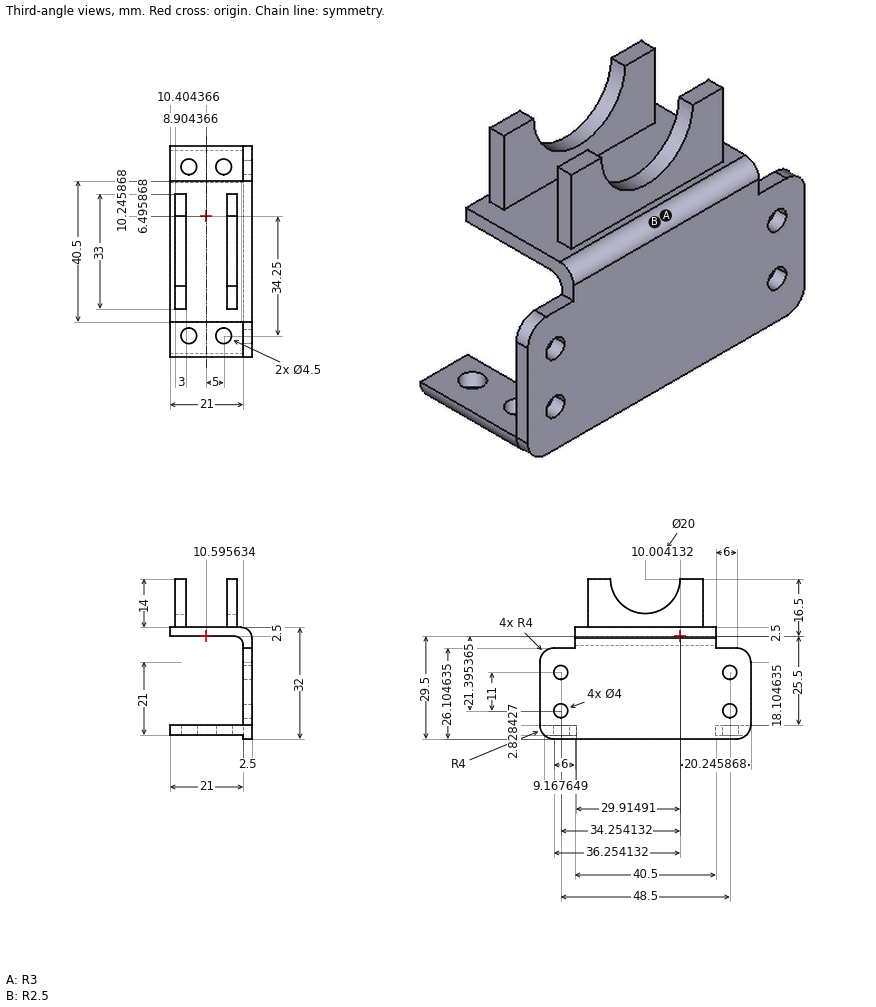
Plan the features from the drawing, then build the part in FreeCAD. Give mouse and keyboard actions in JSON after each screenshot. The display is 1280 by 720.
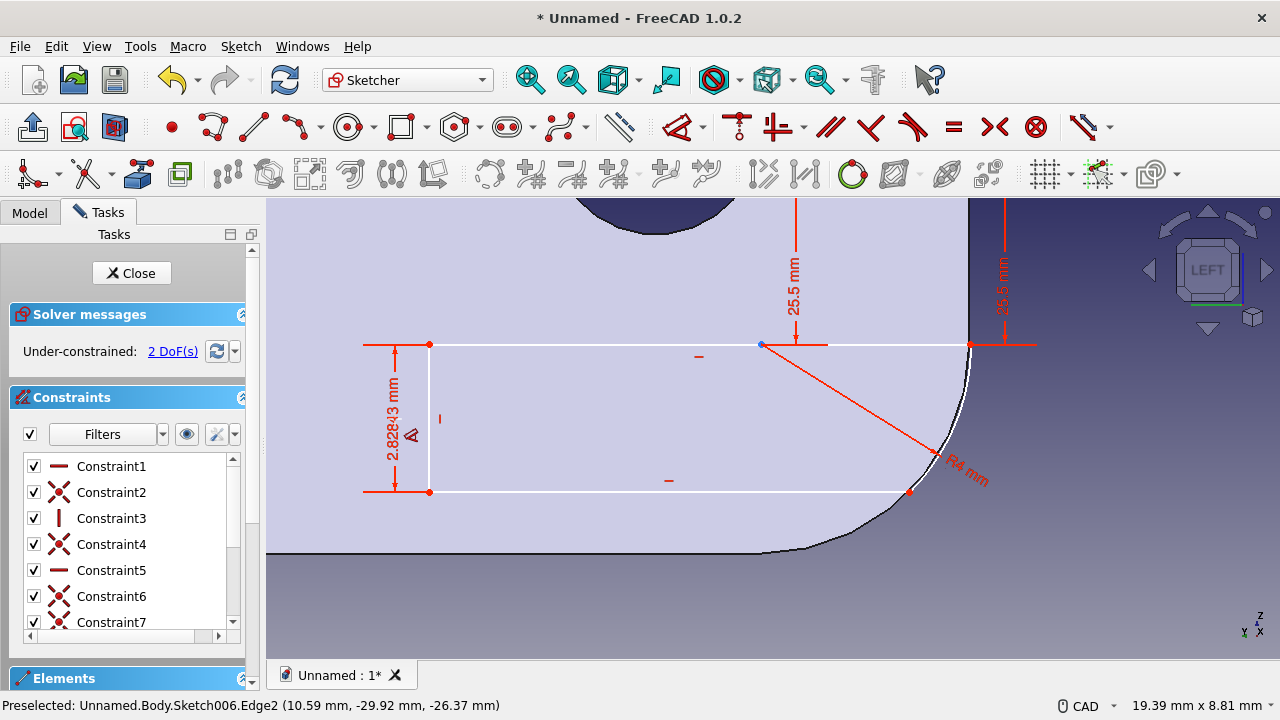
{"action": "left_click", "coordinate": [573, 492]}
{"action": "left_click", "coordinate": [669, 526]}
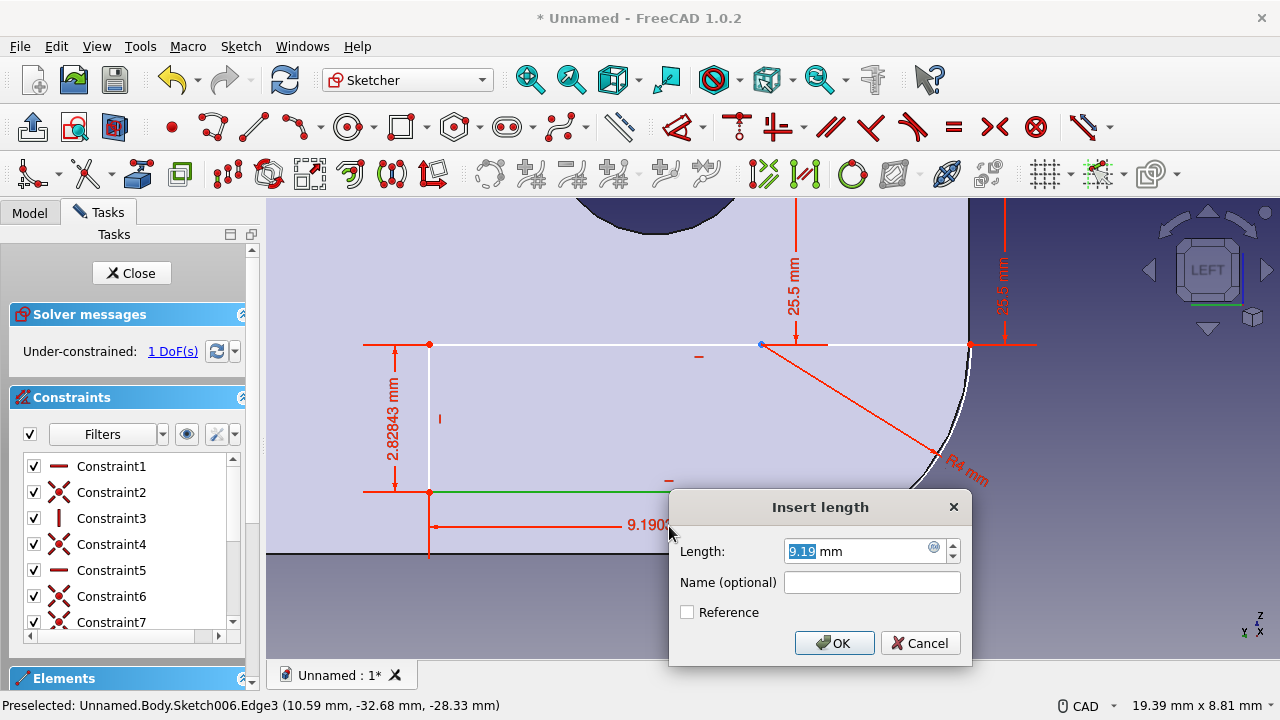
{"action": "type", "text": "9.167649"}
{"action": "key", "text": "Return"}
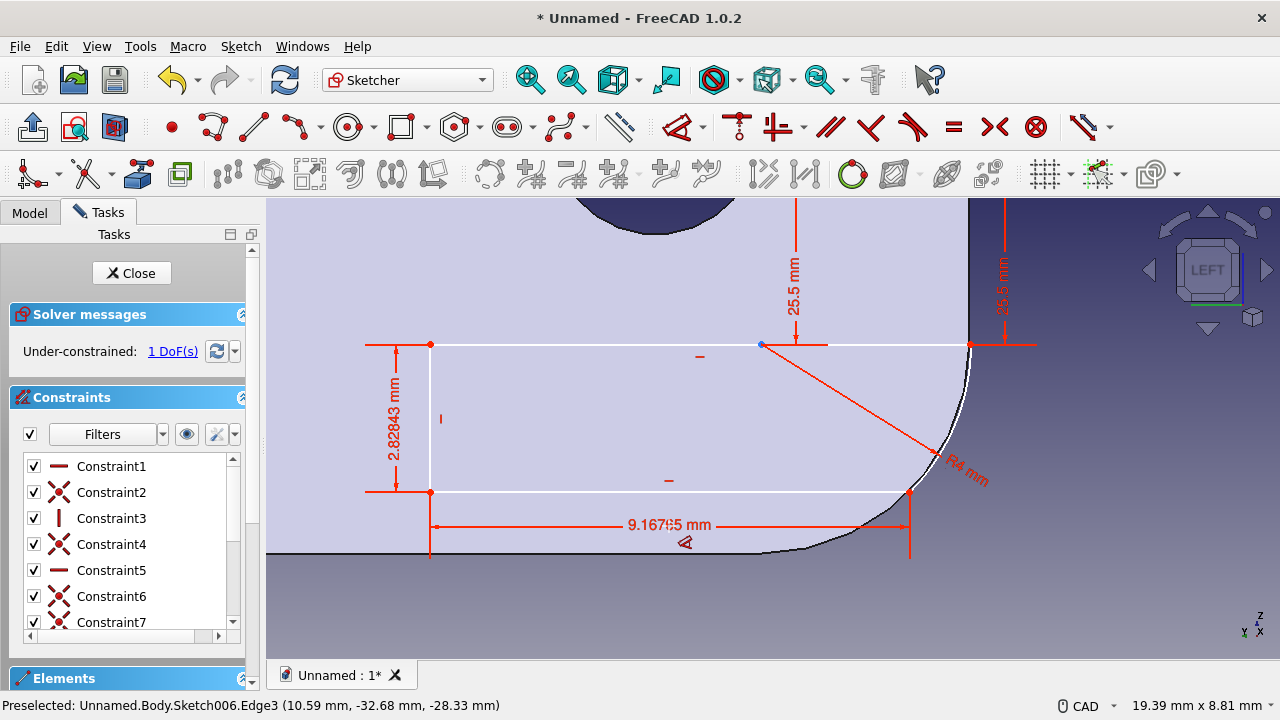
{"action": "left_click", "coordinate": [430, 345]}
{"action": "left_click", "coordinate": [362, 379]}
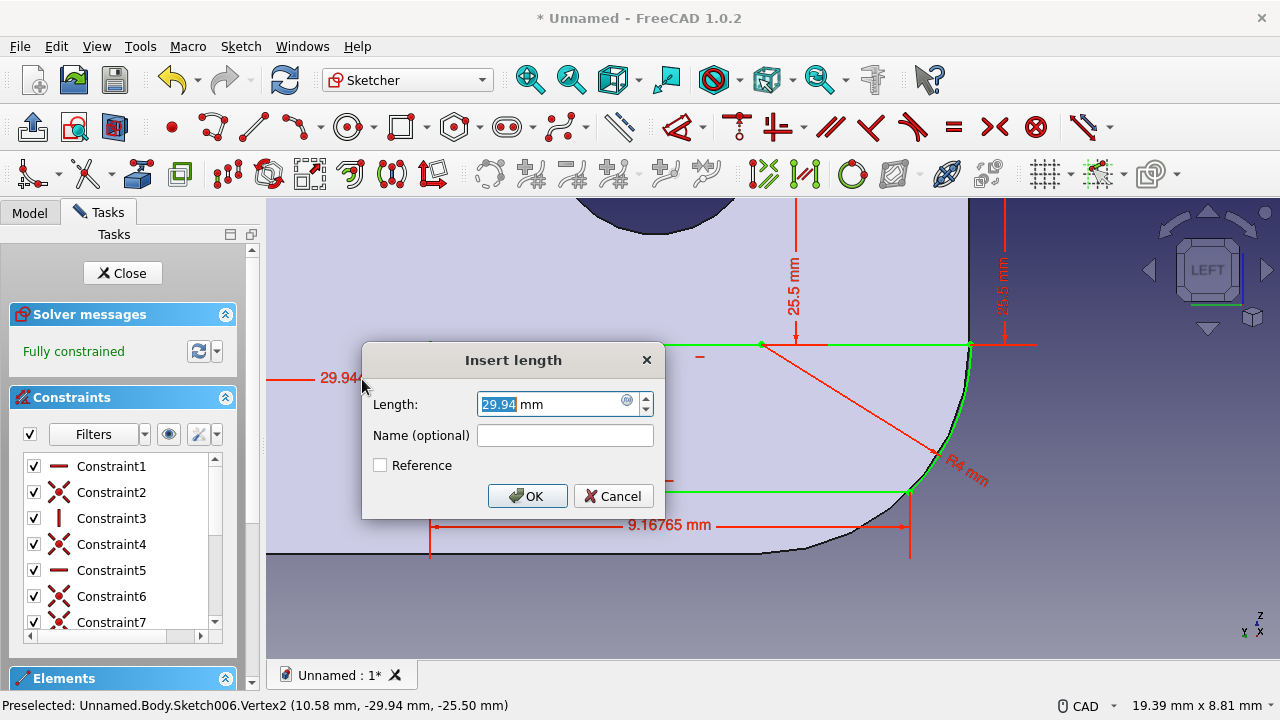
{"action": "type", "text": "29.91491"}
{"action": "key", "text": "Return"}
{"action": "key", "text": "Escape"}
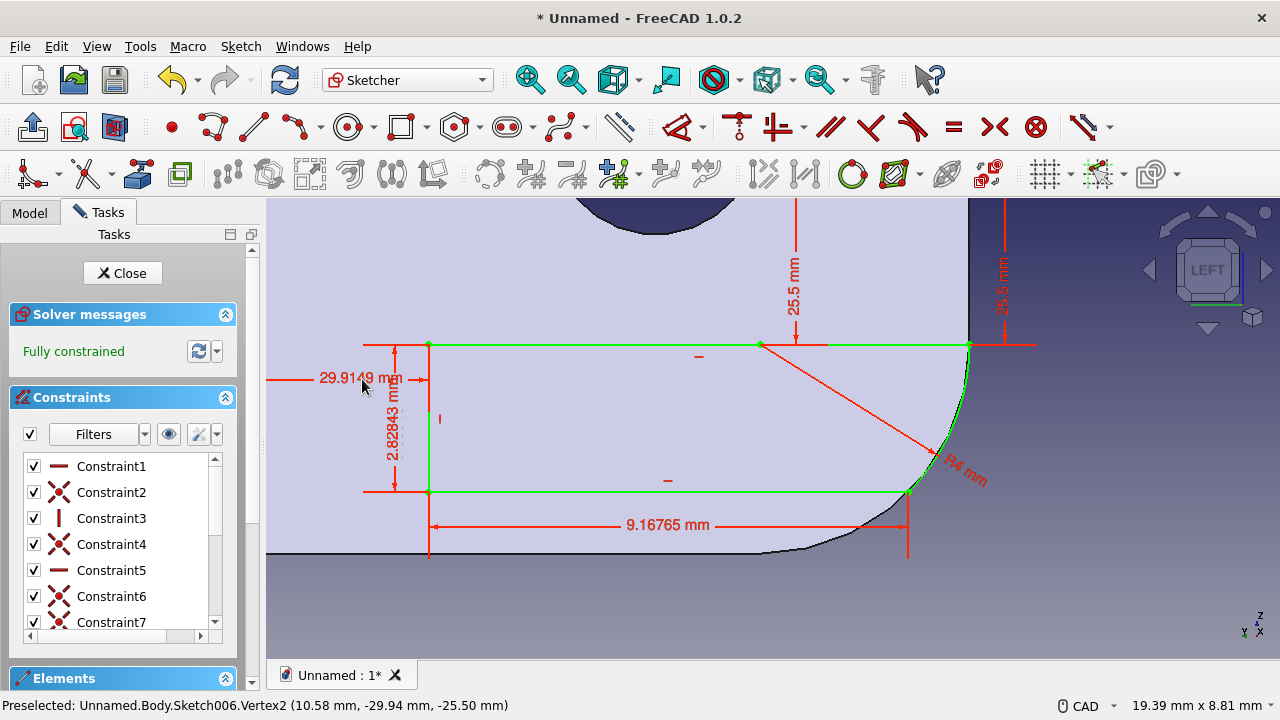
{"action": "left_click", "coordinate": [123, 273]}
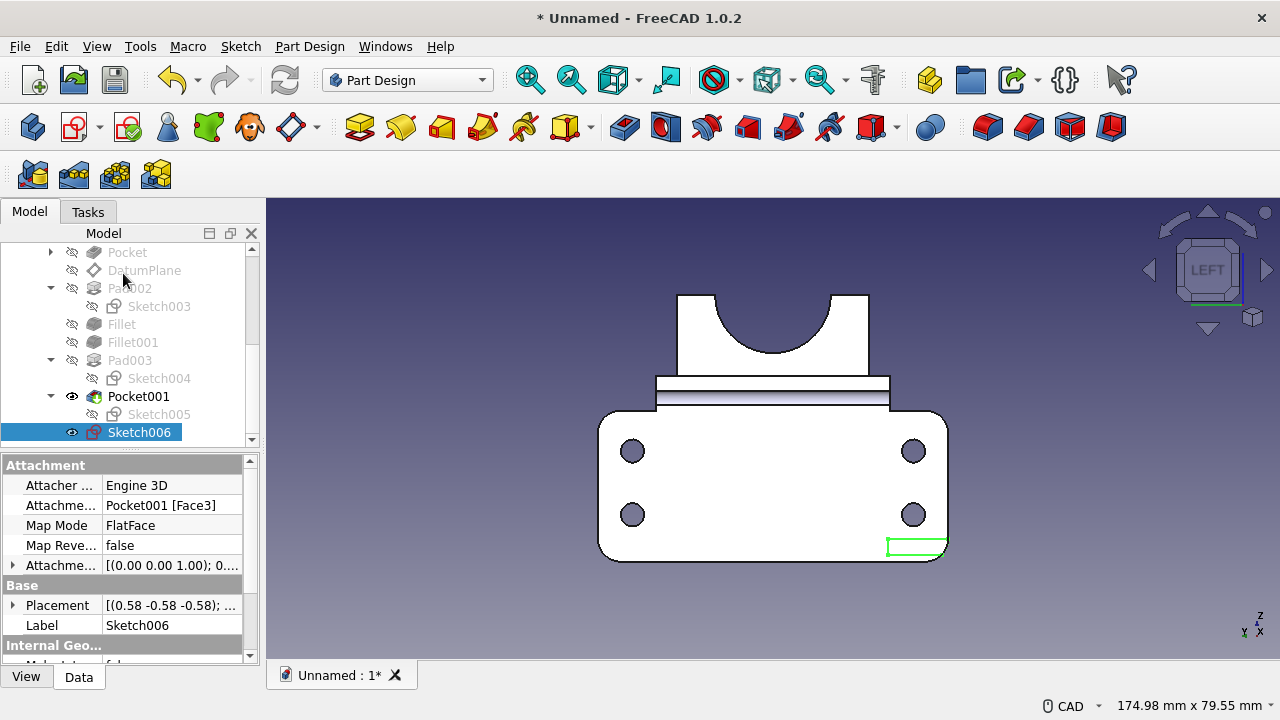
{"action": "left_click", "coordinate": [360, 128]}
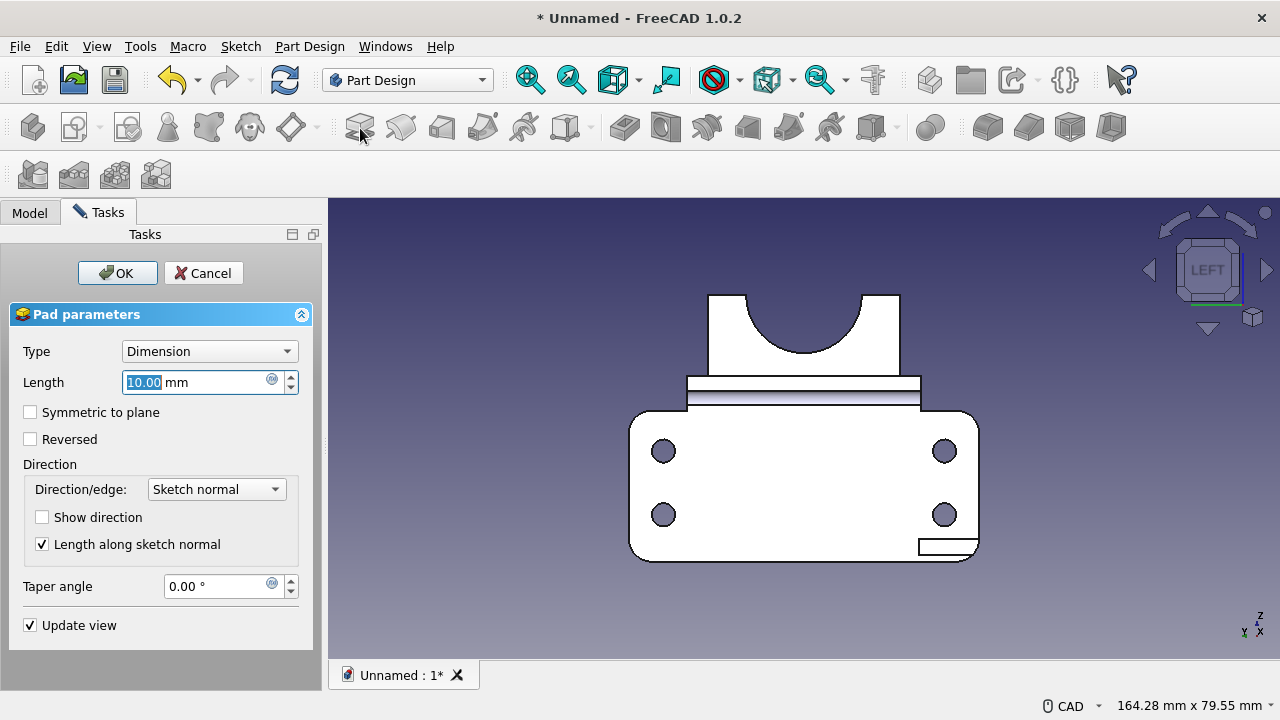
{"action": "type", "text": "21"}
{"action": "key", "text": "Tab"}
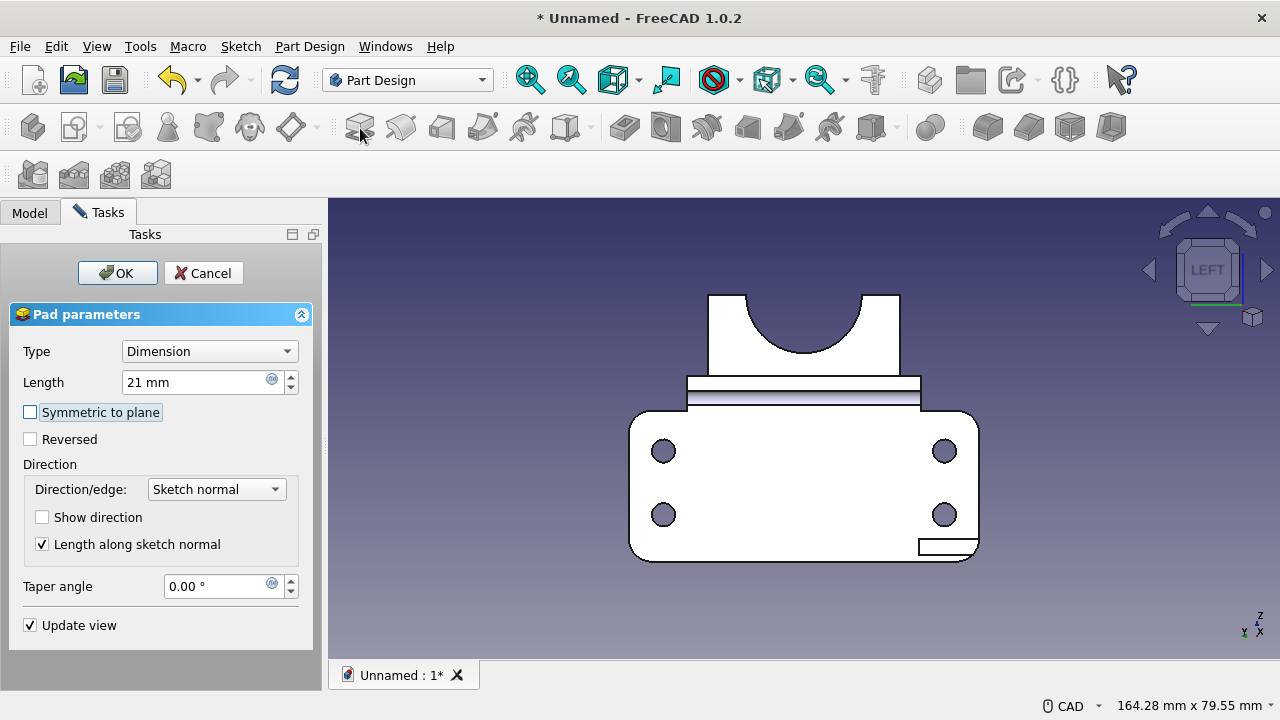
{"action": "left_click", "coordinate": [118, 273]}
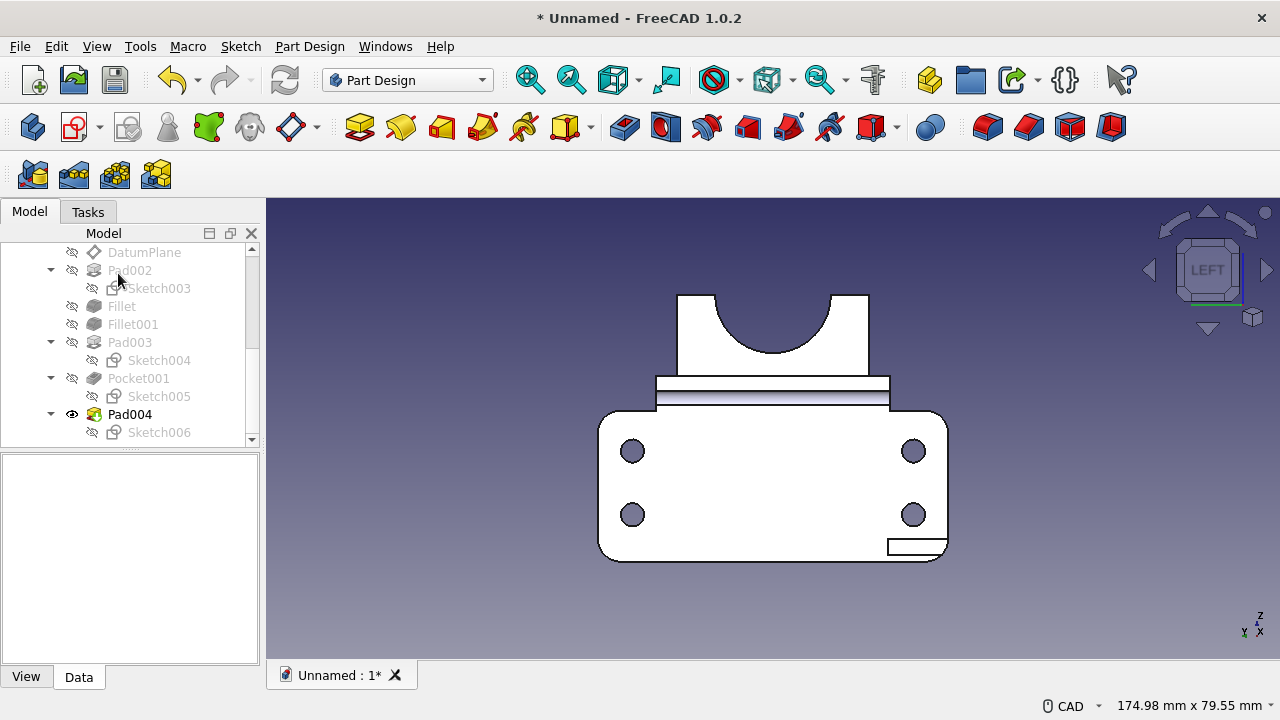
{"action": "scroll", "coordinate": [141, 338], "scroll_direction": "down", "scroll_amount": 3}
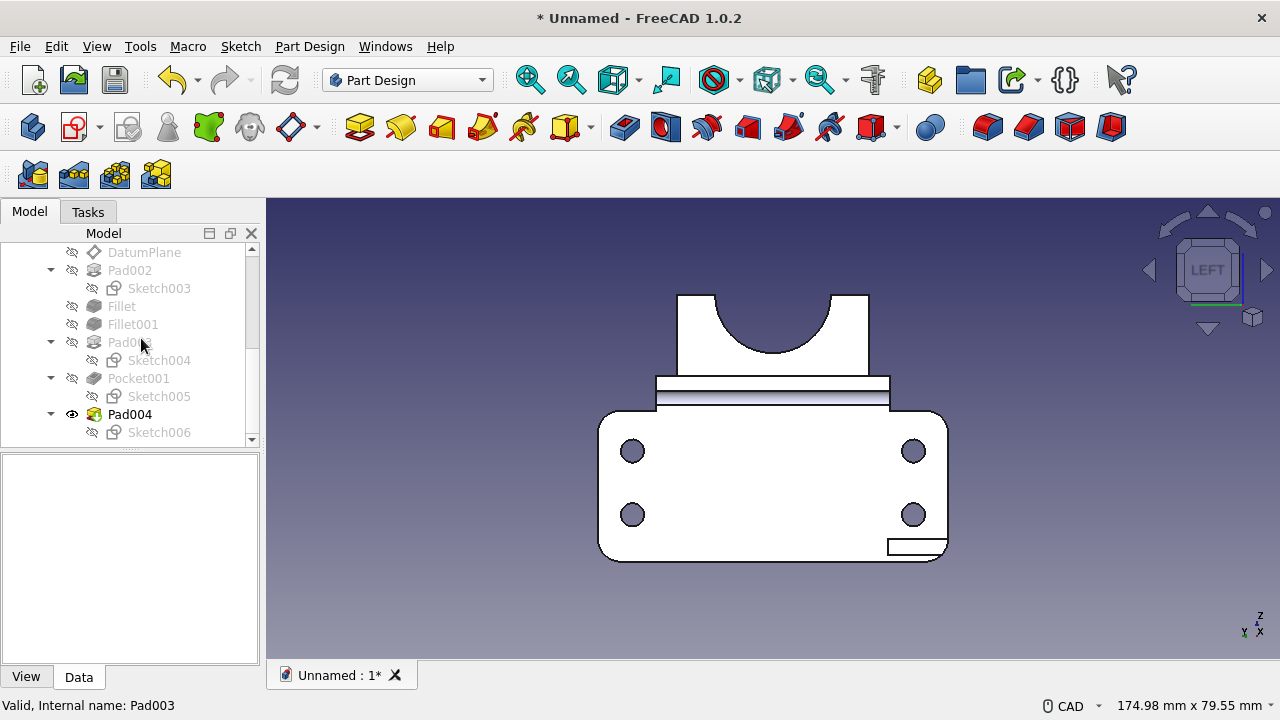
{"action": "scroll", "coordinate": [141, 338], "scroll_direction": "up", "scroll_amount": 15}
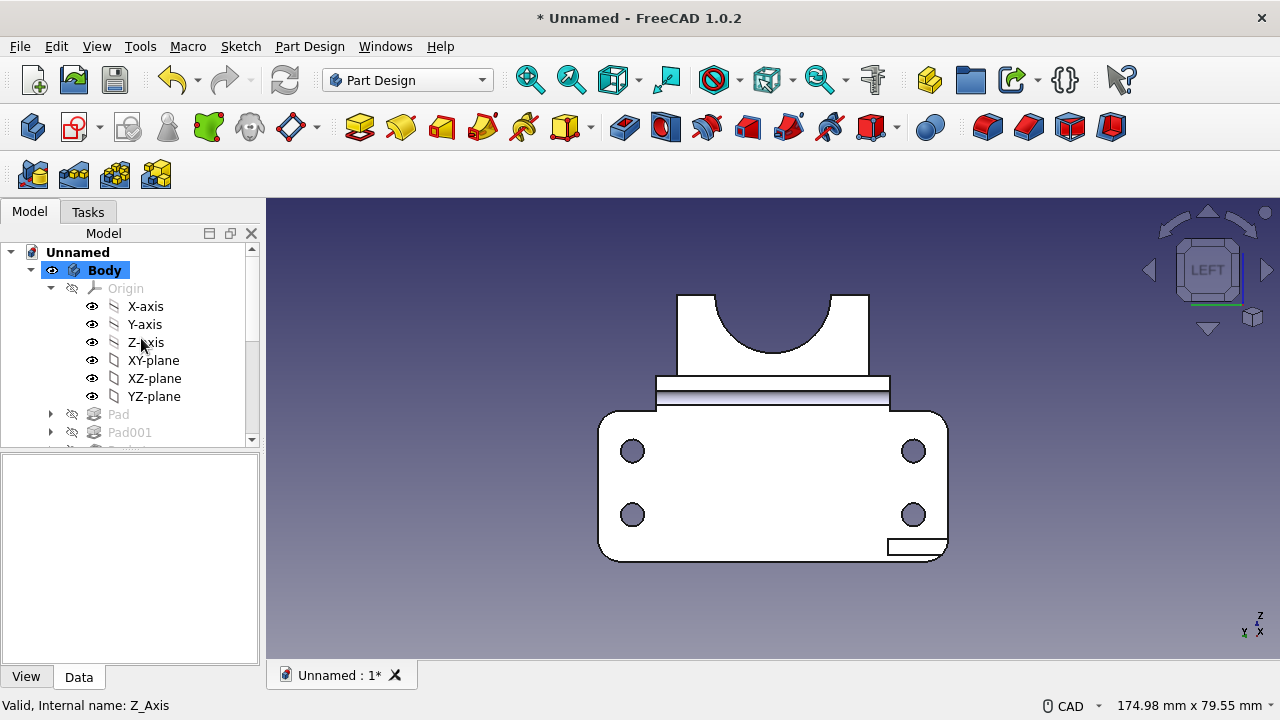
{"action": "left_click", "coordinate": [137, 378]}